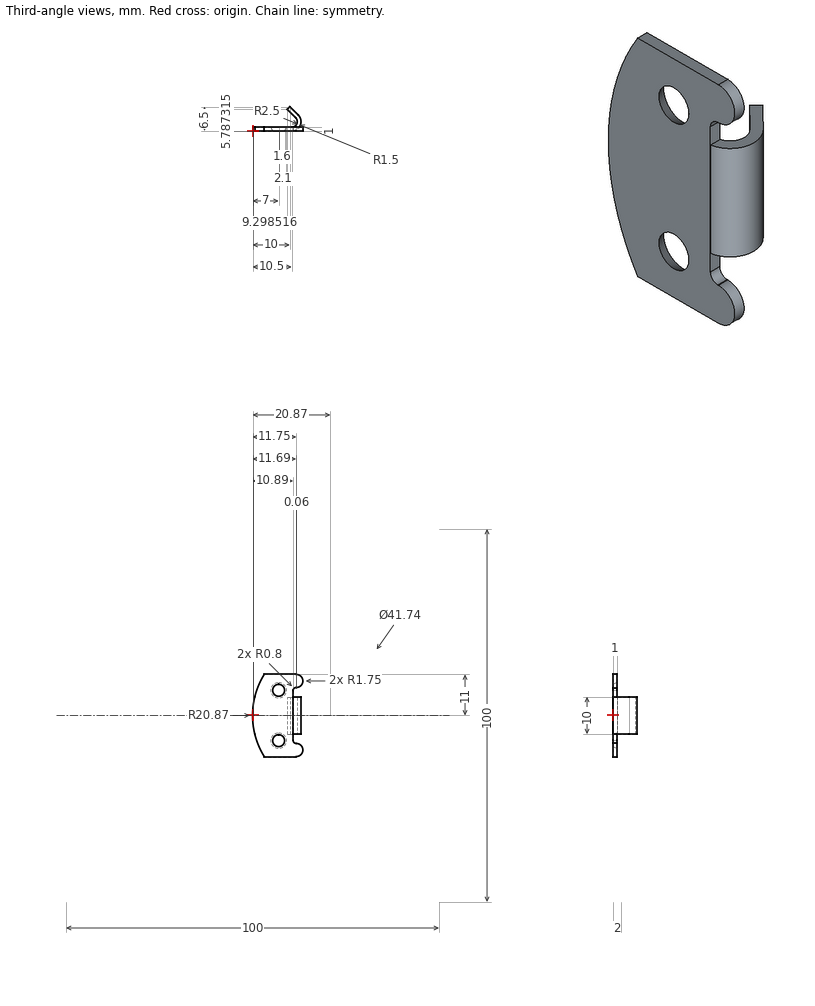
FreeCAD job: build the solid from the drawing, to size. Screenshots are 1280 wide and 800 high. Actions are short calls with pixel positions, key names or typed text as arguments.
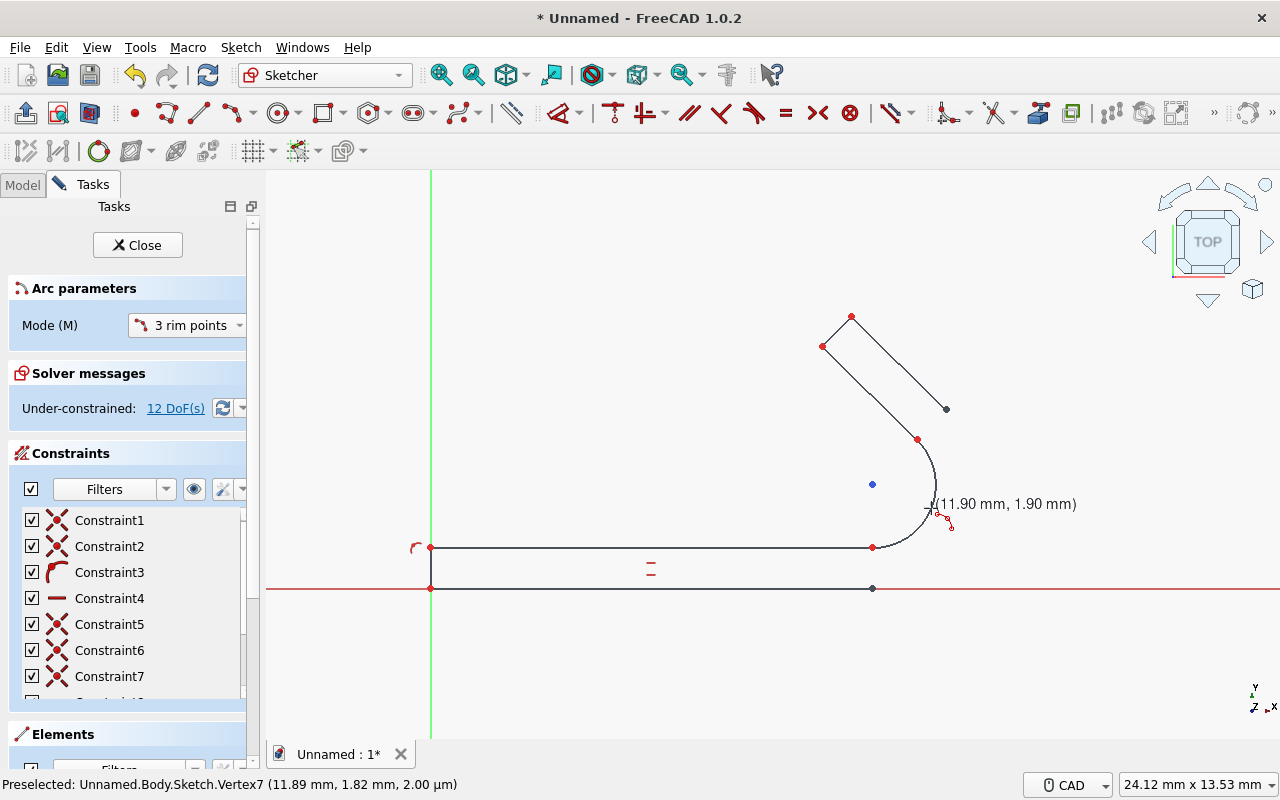
click(872, 589)
click(946, 410)
click(970, 524)
key(Escape)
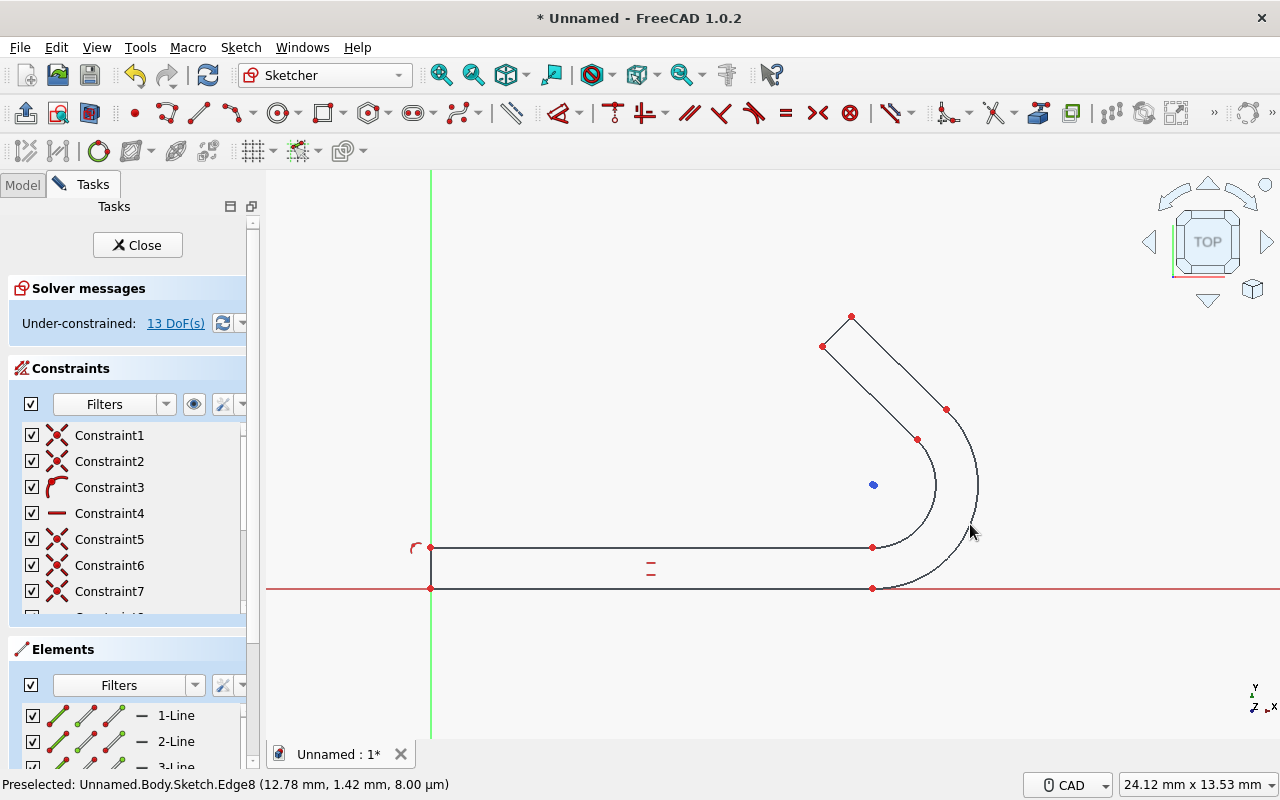
click(918, 382)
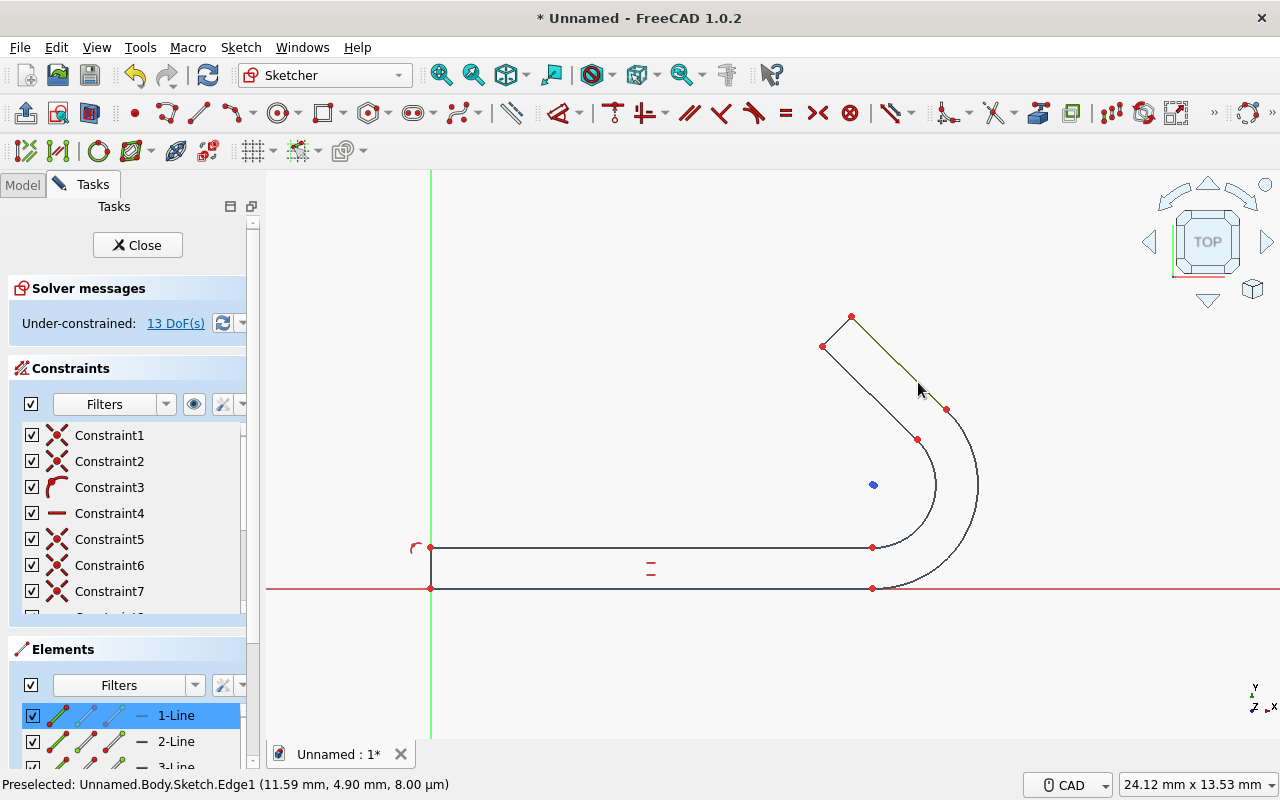
click(941, 565)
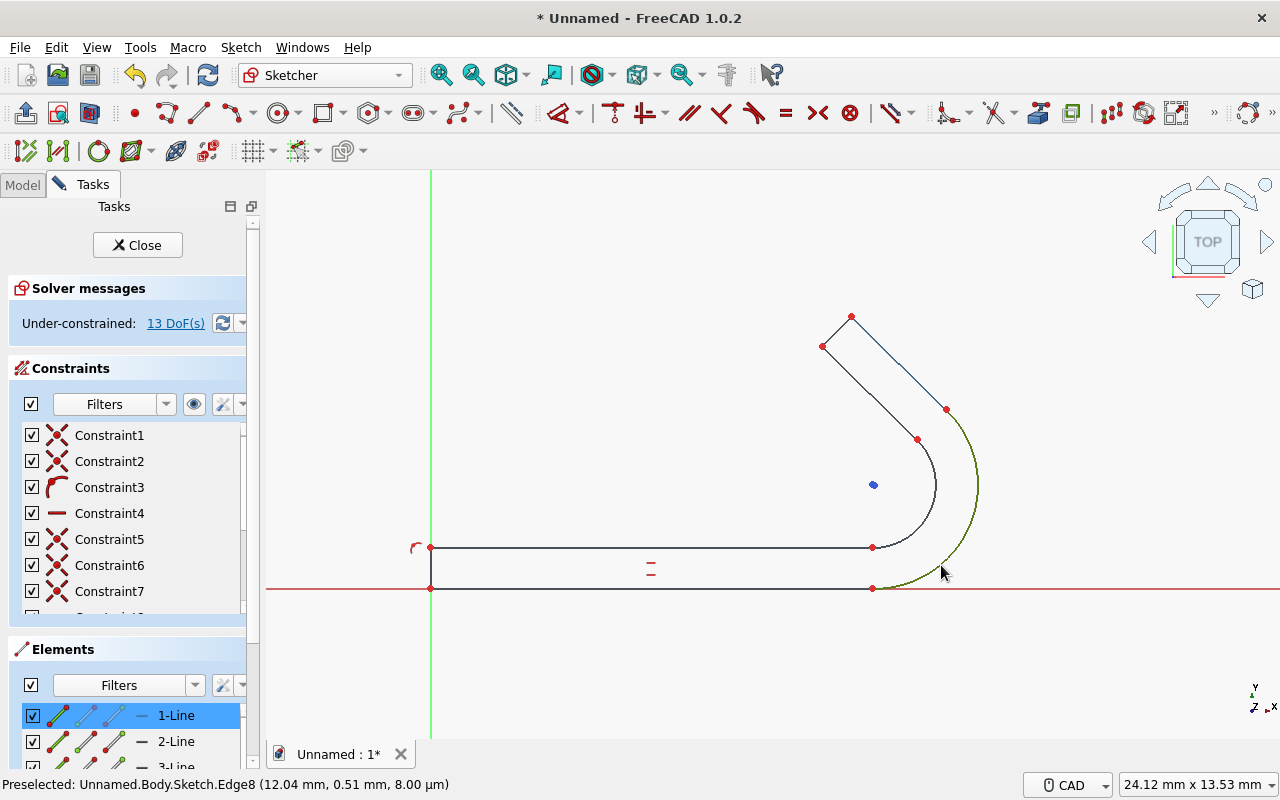
click(754, 114)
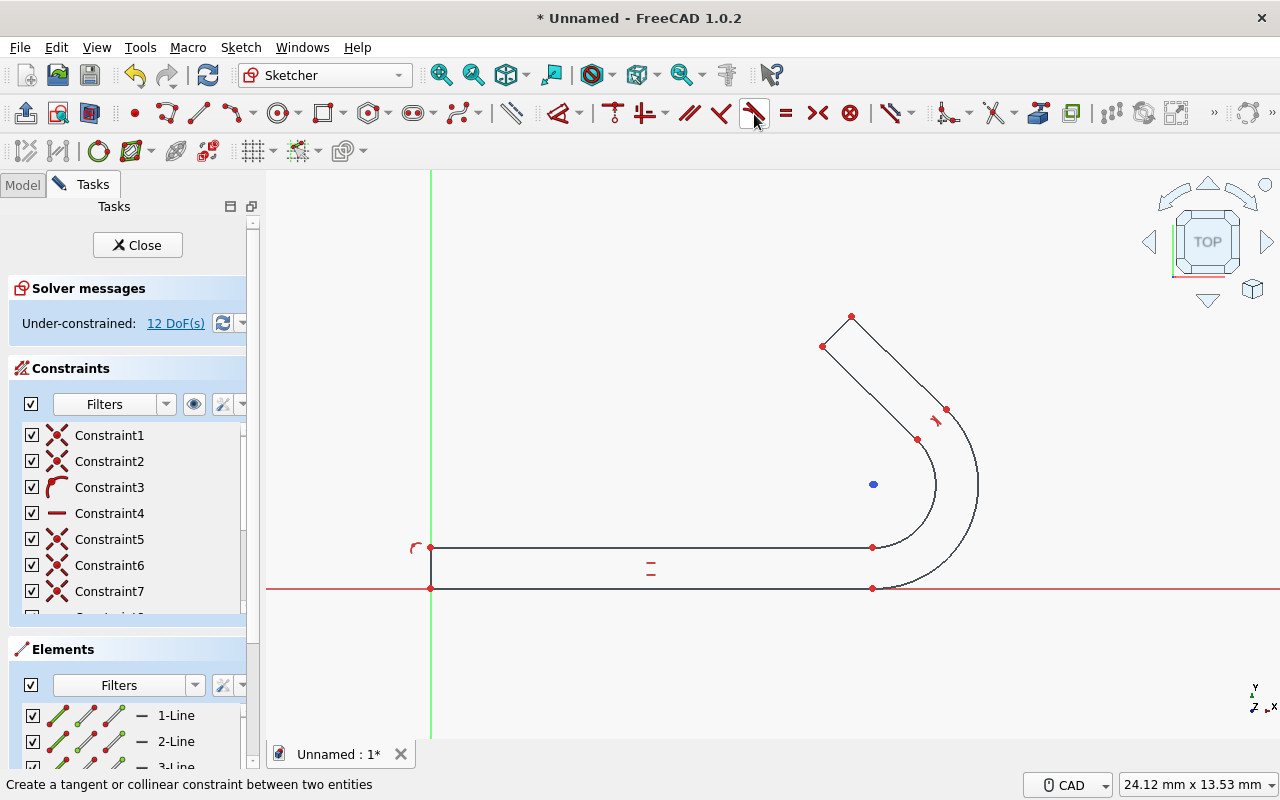
click(850, 375)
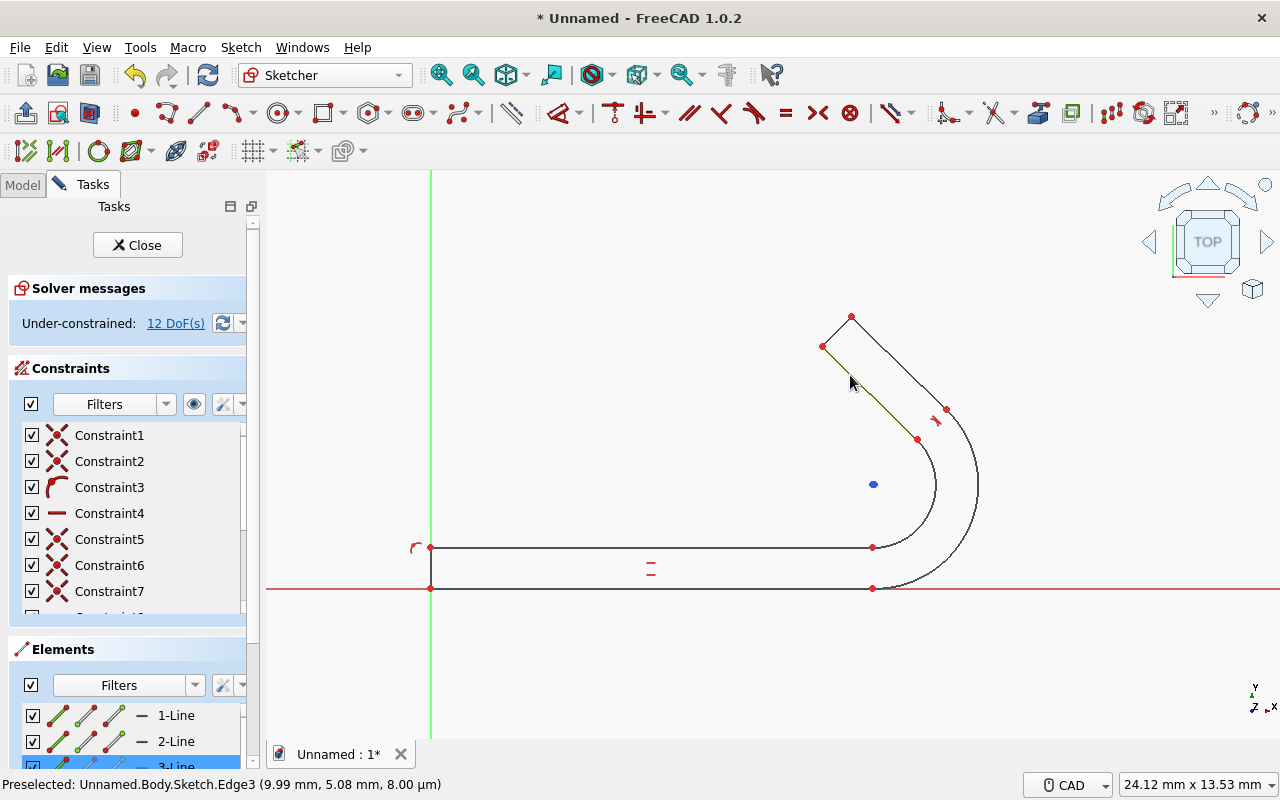
click(913, 533)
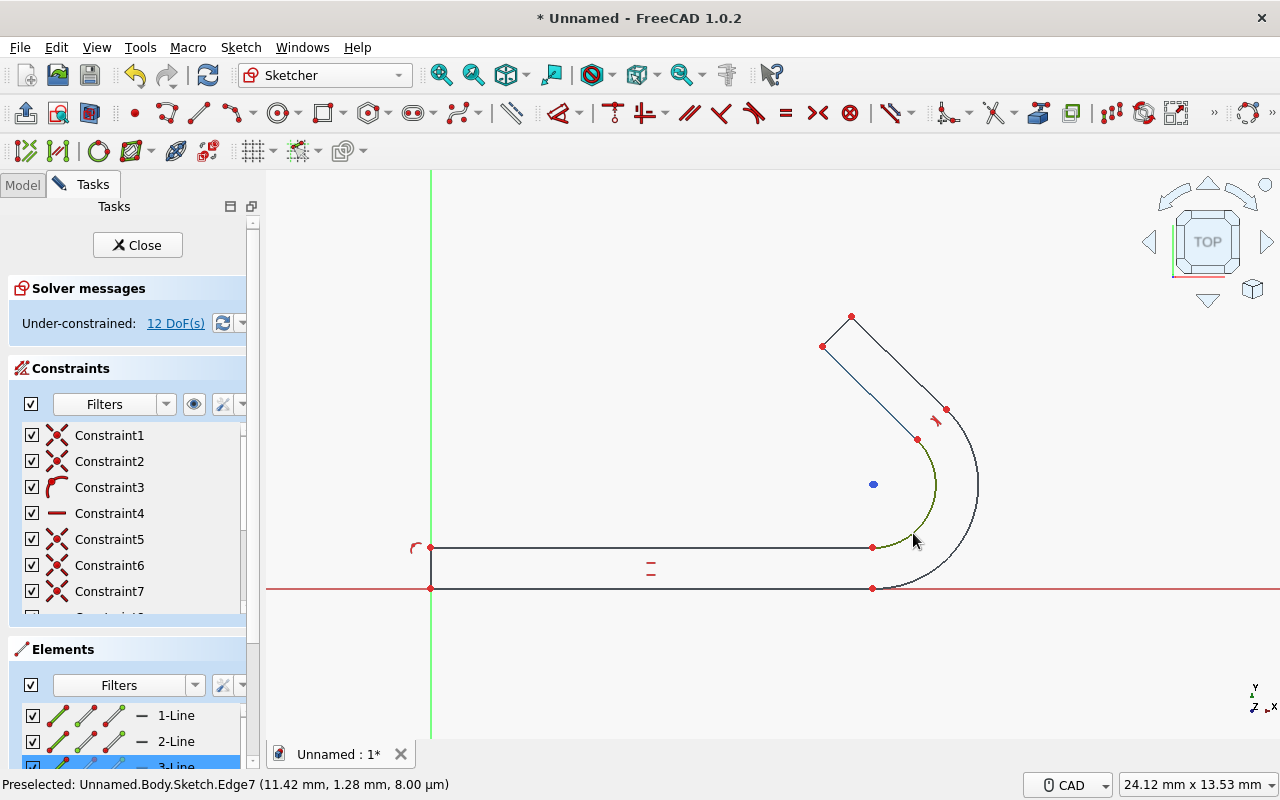
click(754, 114)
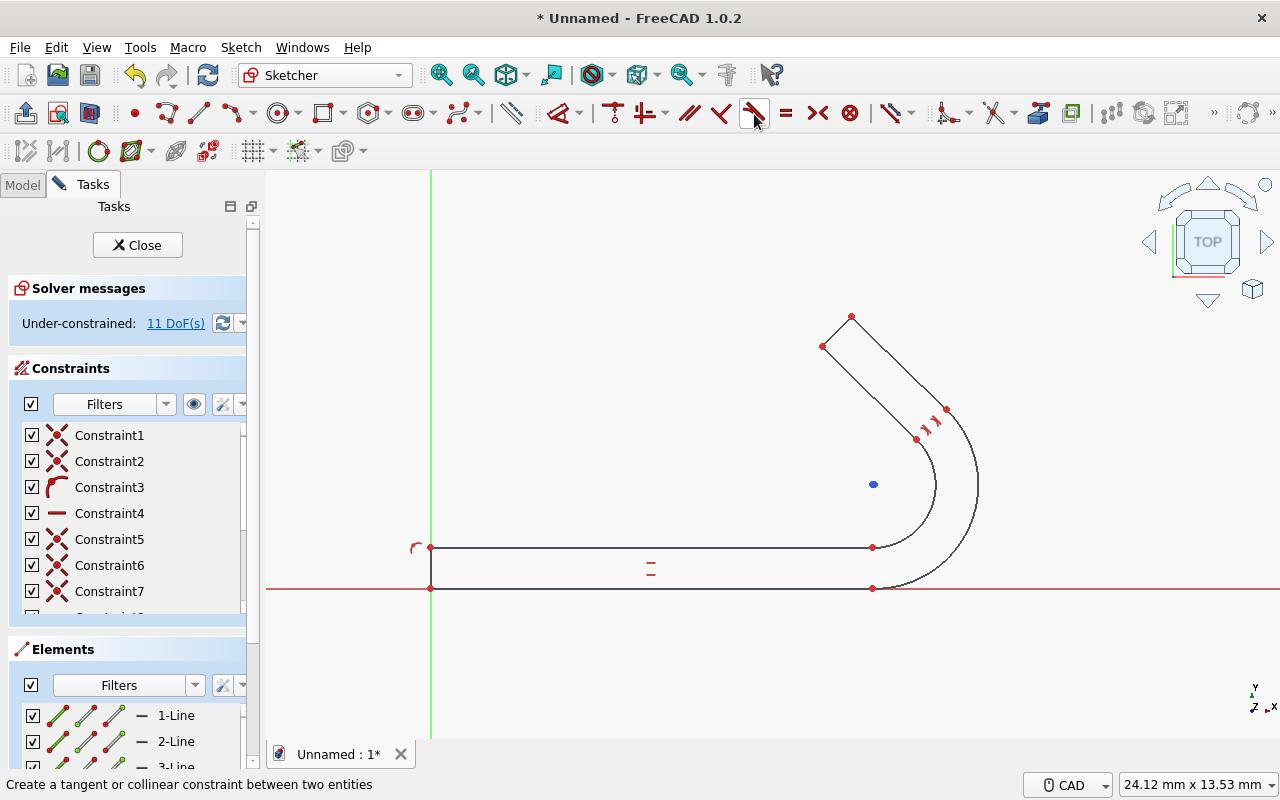
click(740, 548)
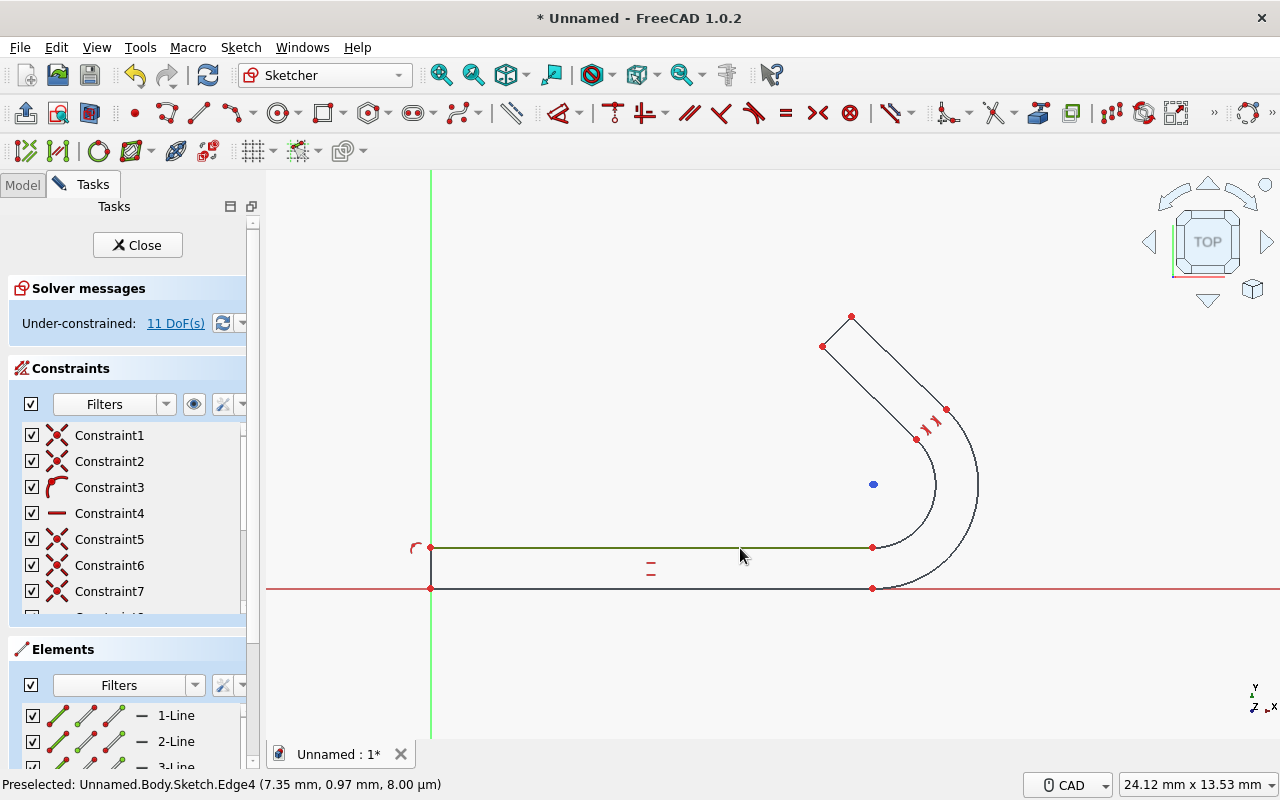
click(913, 533)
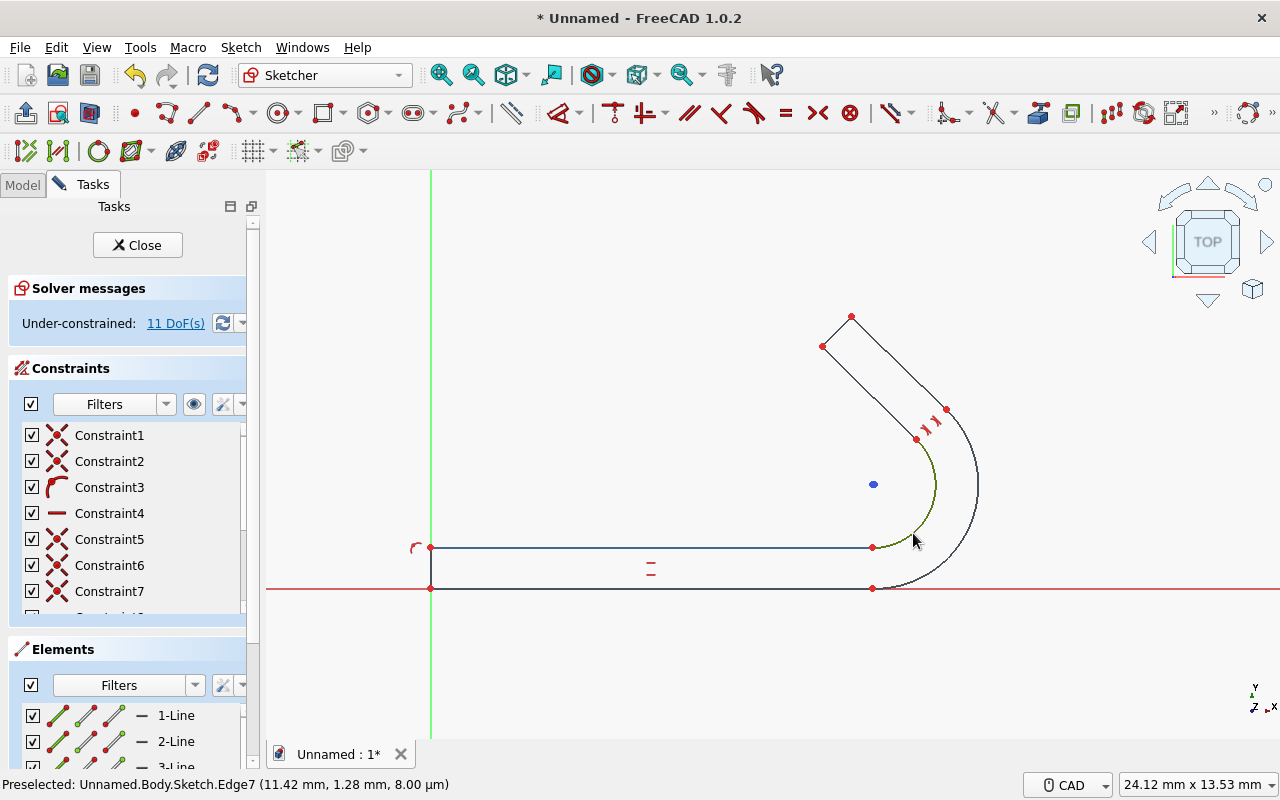
click(754, 114)